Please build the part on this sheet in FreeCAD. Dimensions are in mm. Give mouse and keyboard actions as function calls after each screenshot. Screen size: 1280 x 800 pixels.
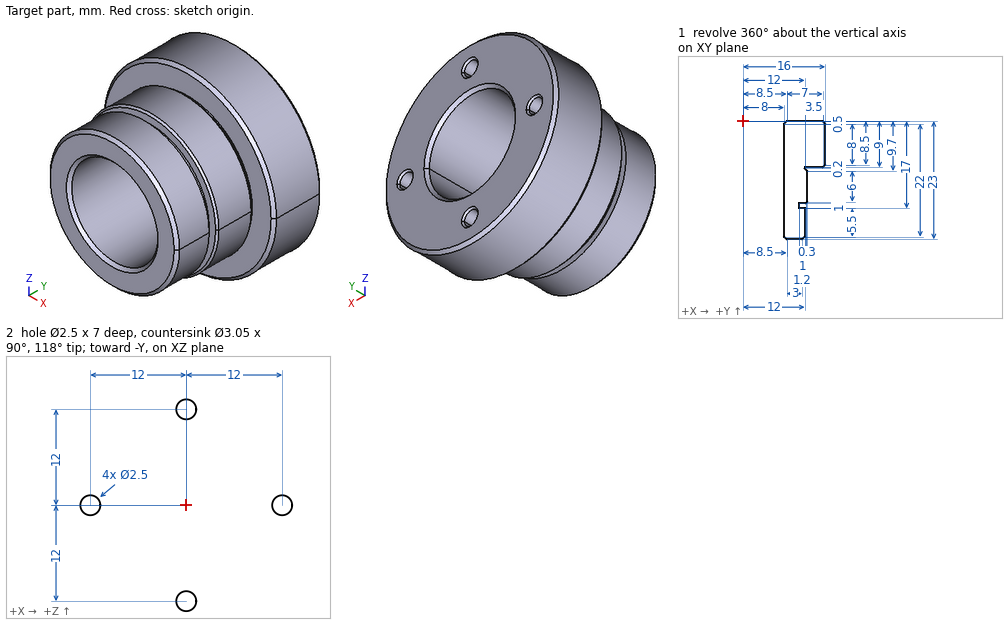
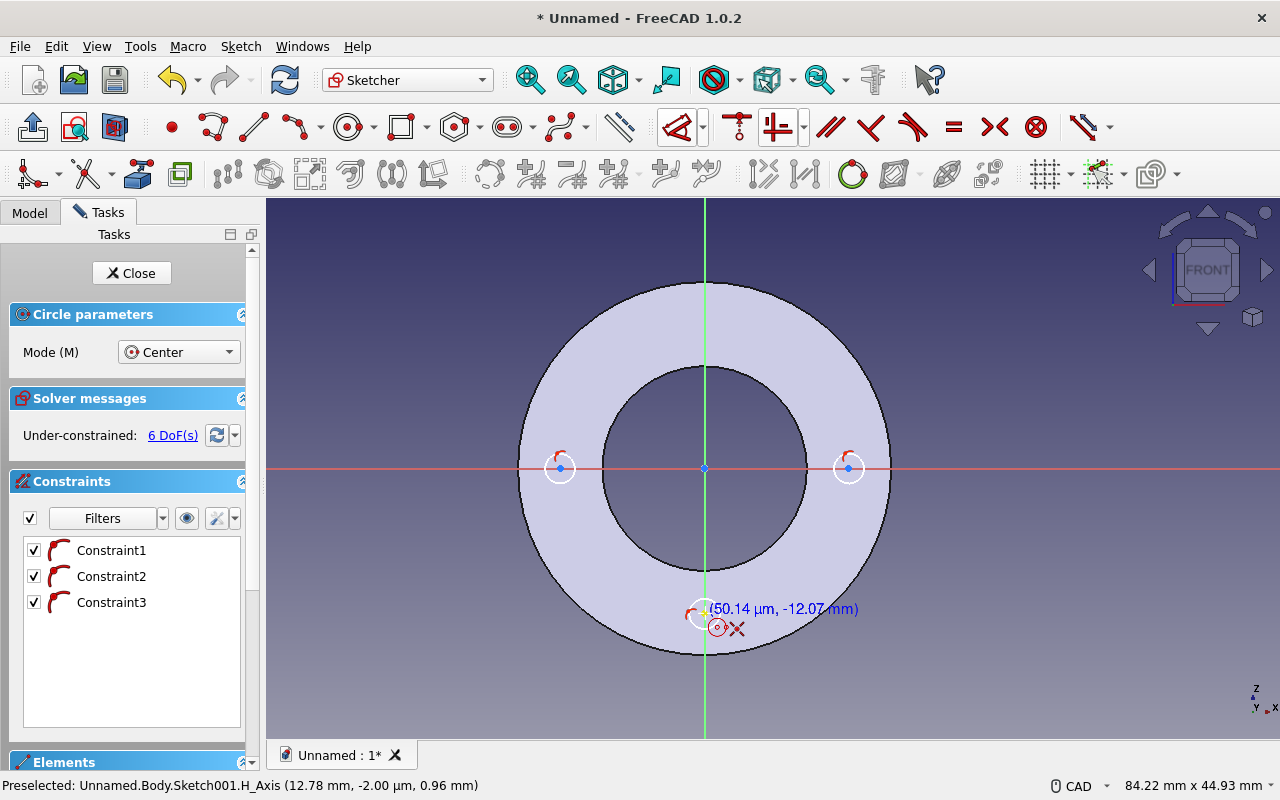
scroll(705, 324, up, 3)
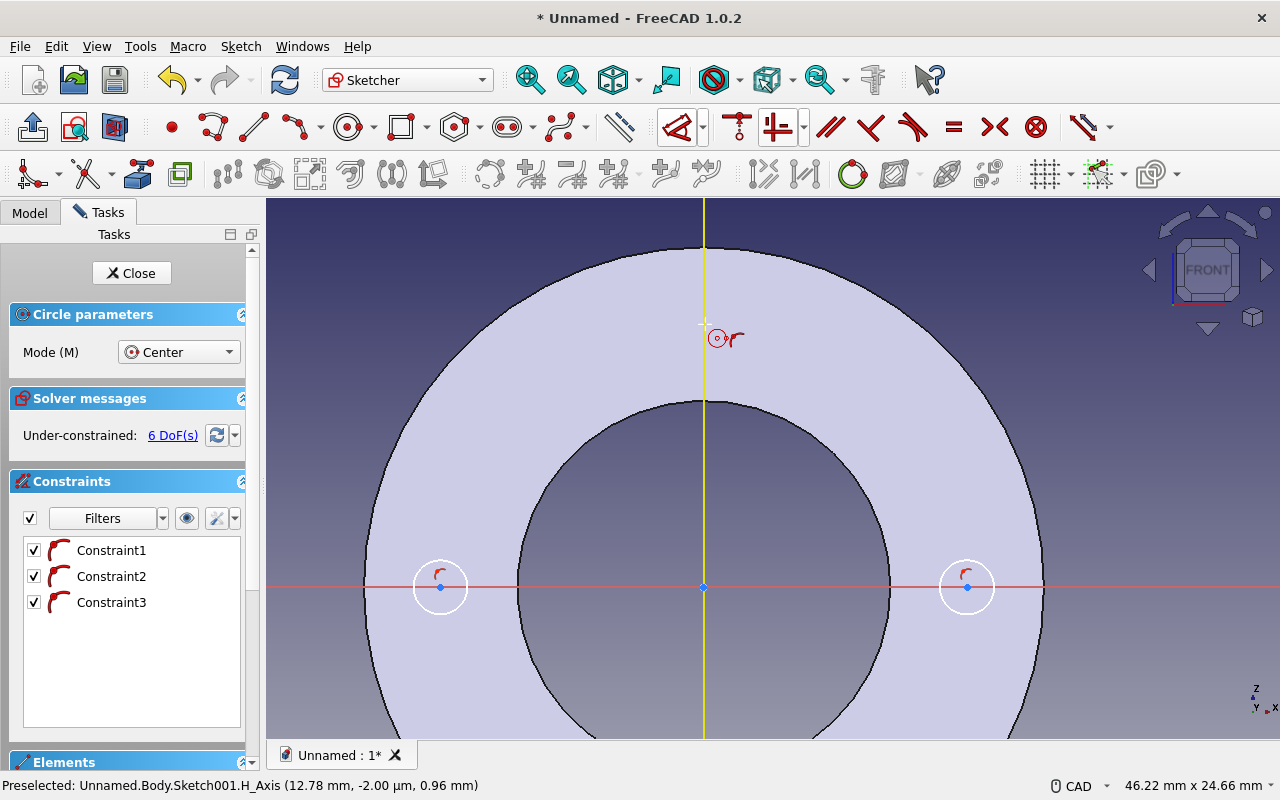
click(704, 324)
click(723, 305)
key(Escape)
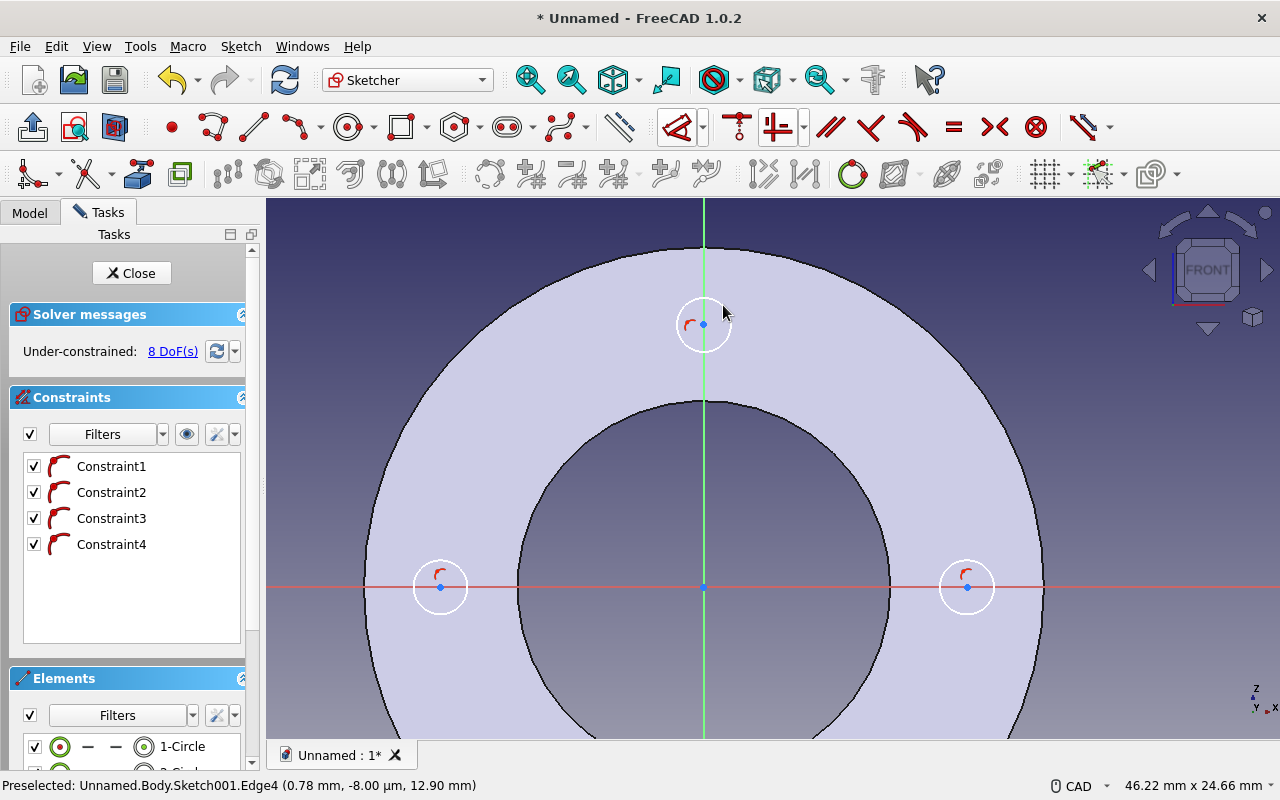
click(460, 568)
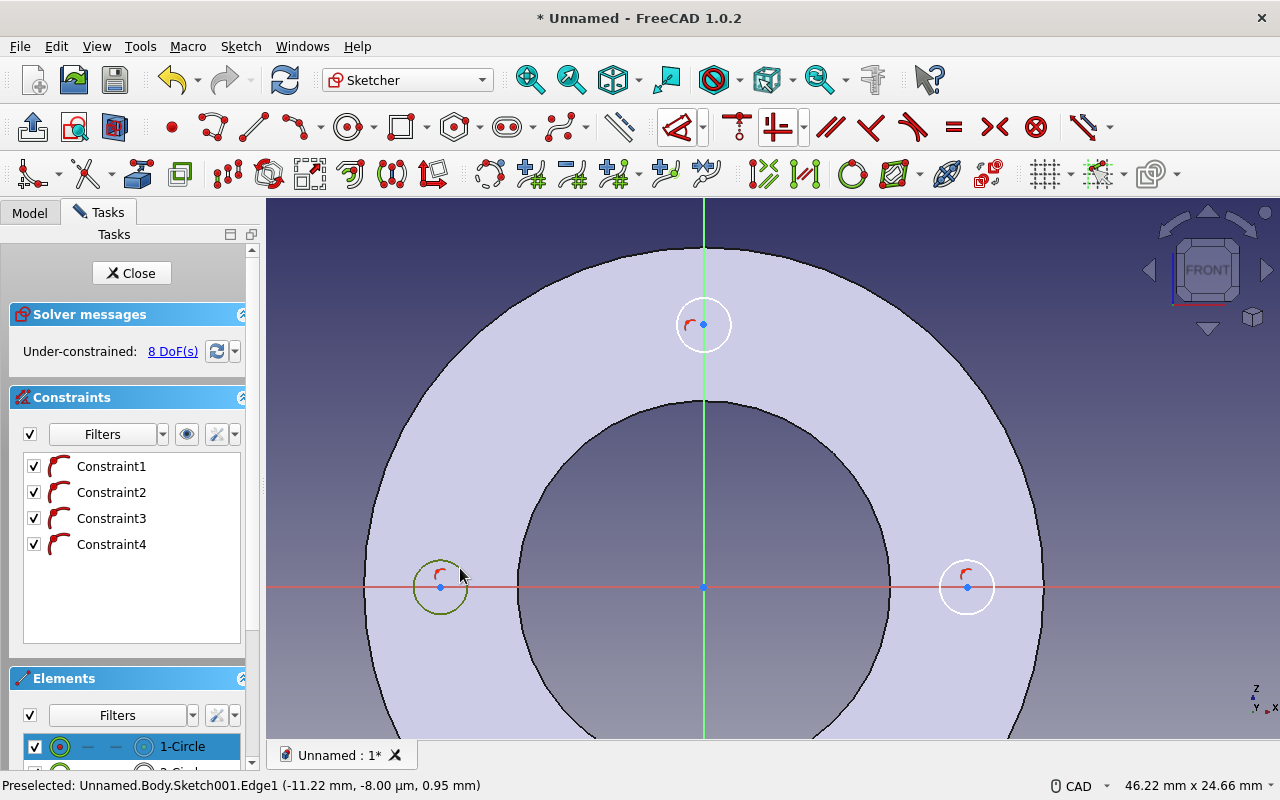
scroll(705, 324, down, 3)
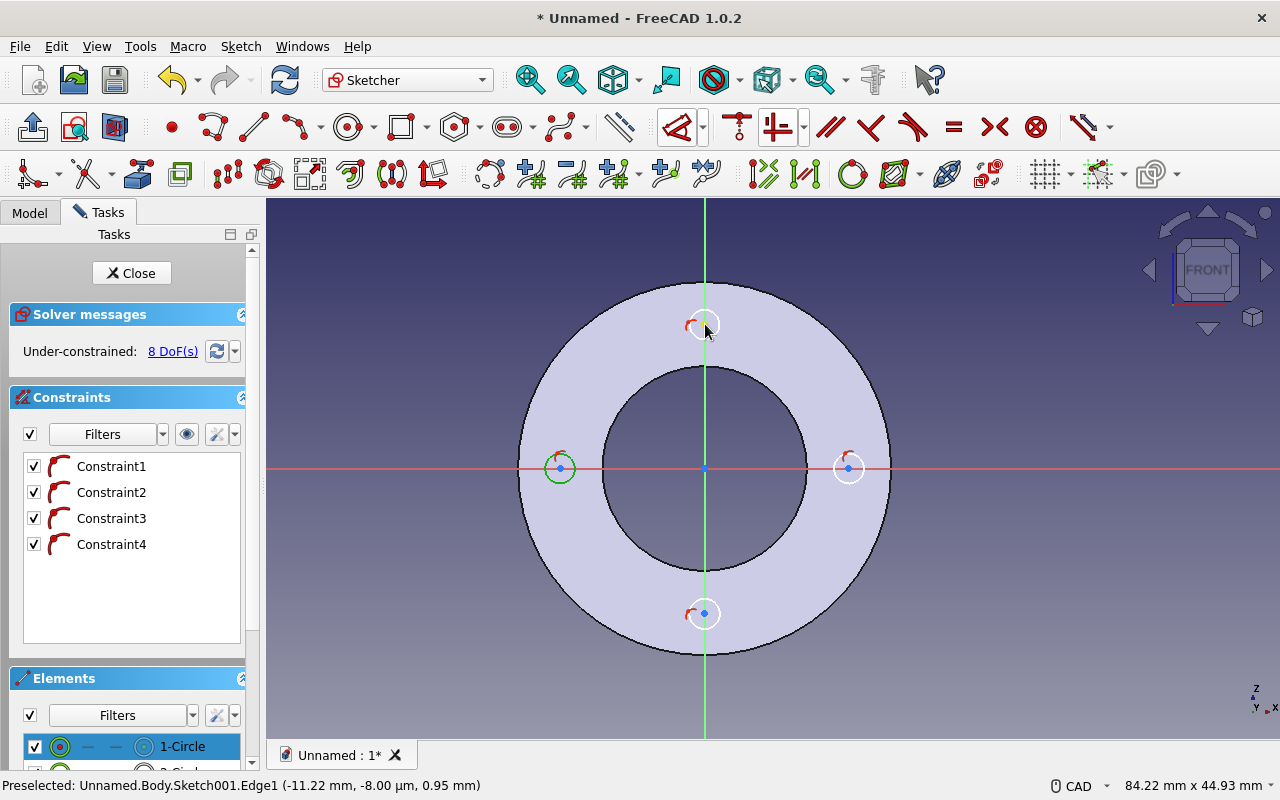
scroll(715, 603, up, 2)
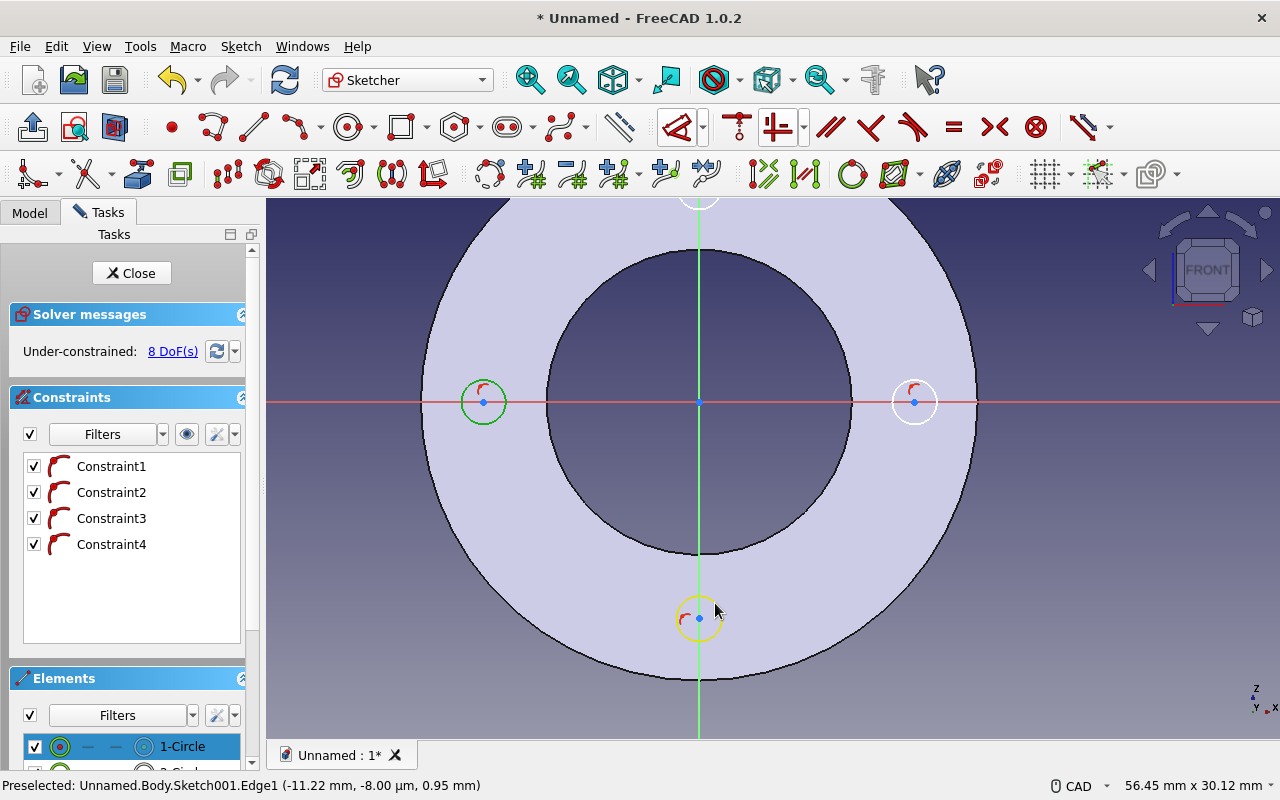
click(715, 603)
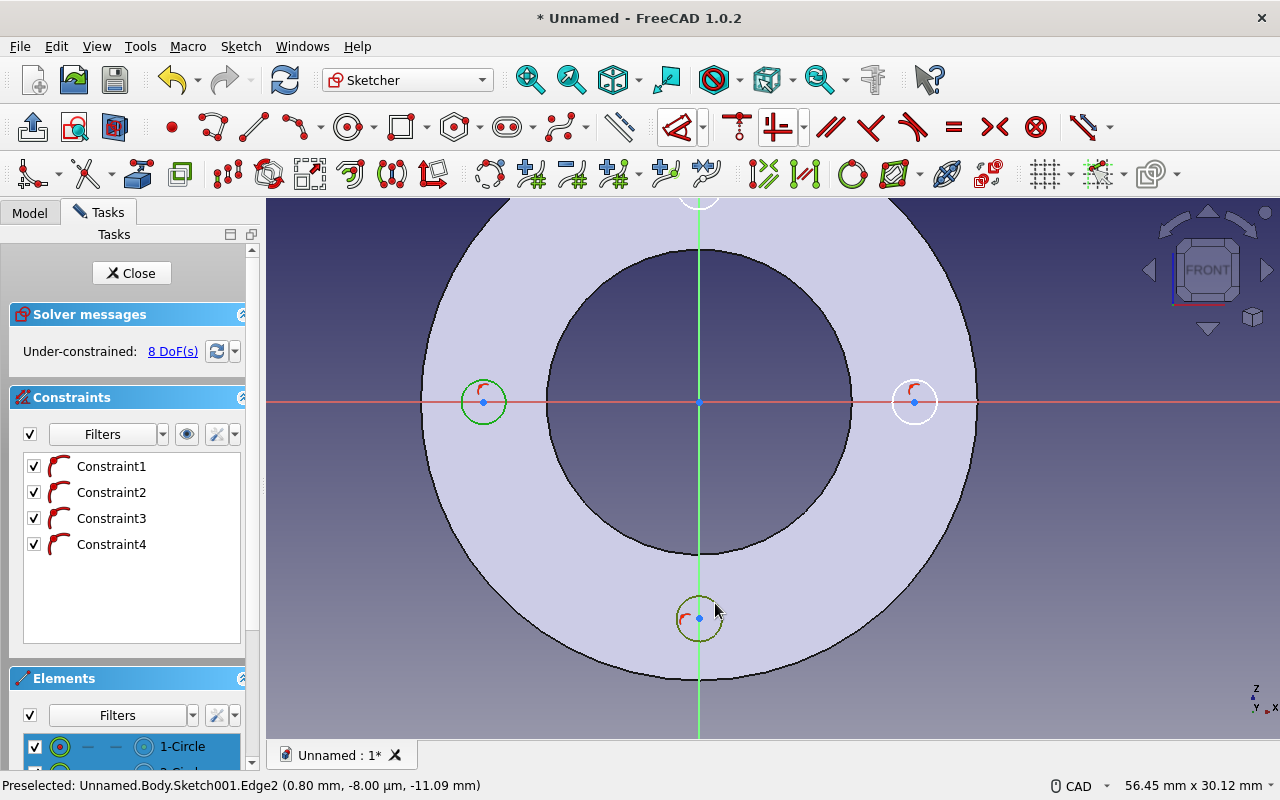
click(930, 386)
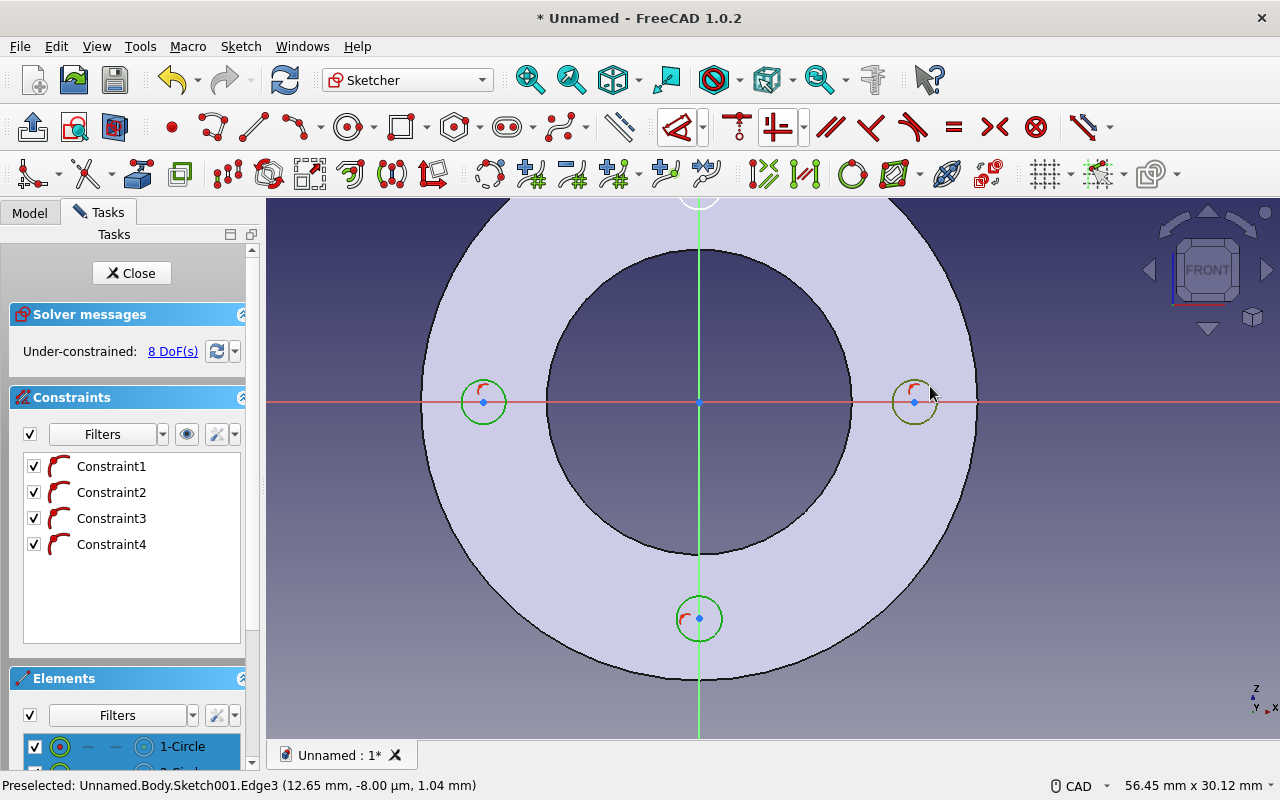
scroll(715, 603, down, 2)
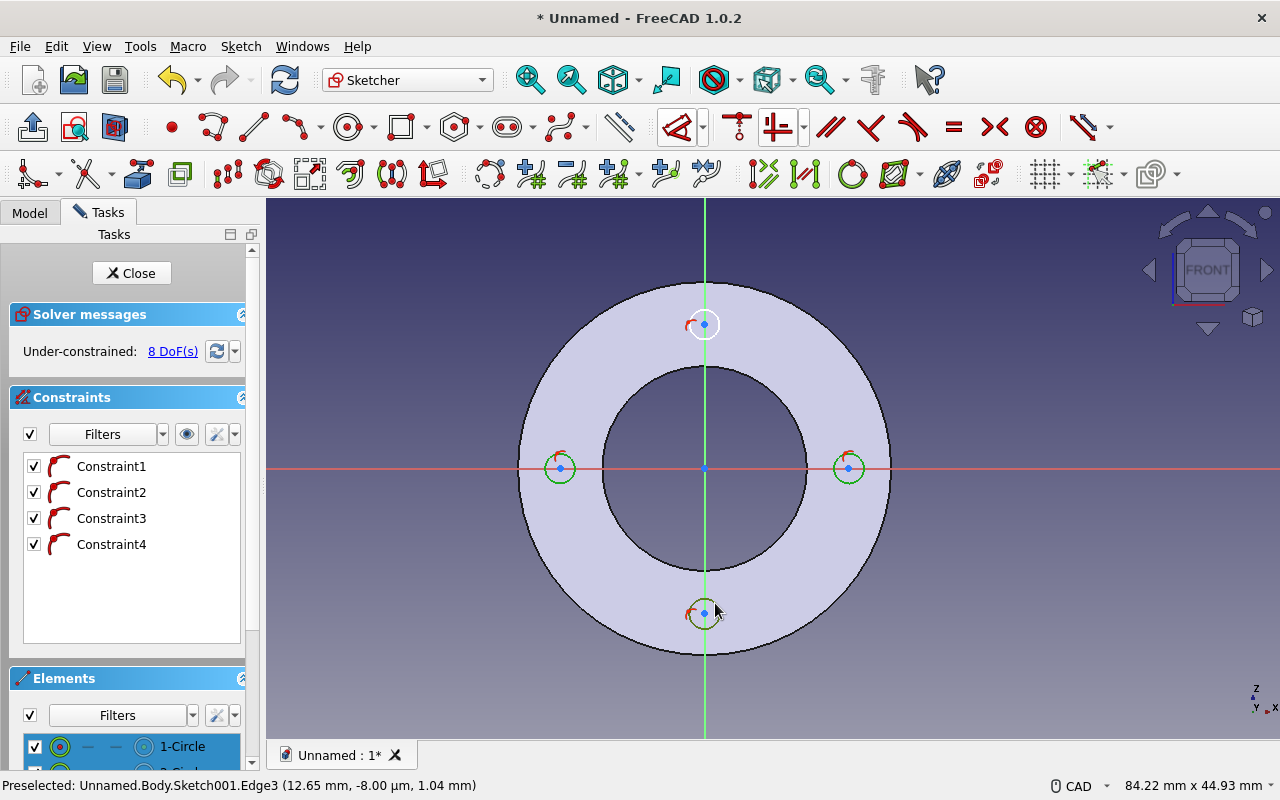
scroll(715, 314, up, 2)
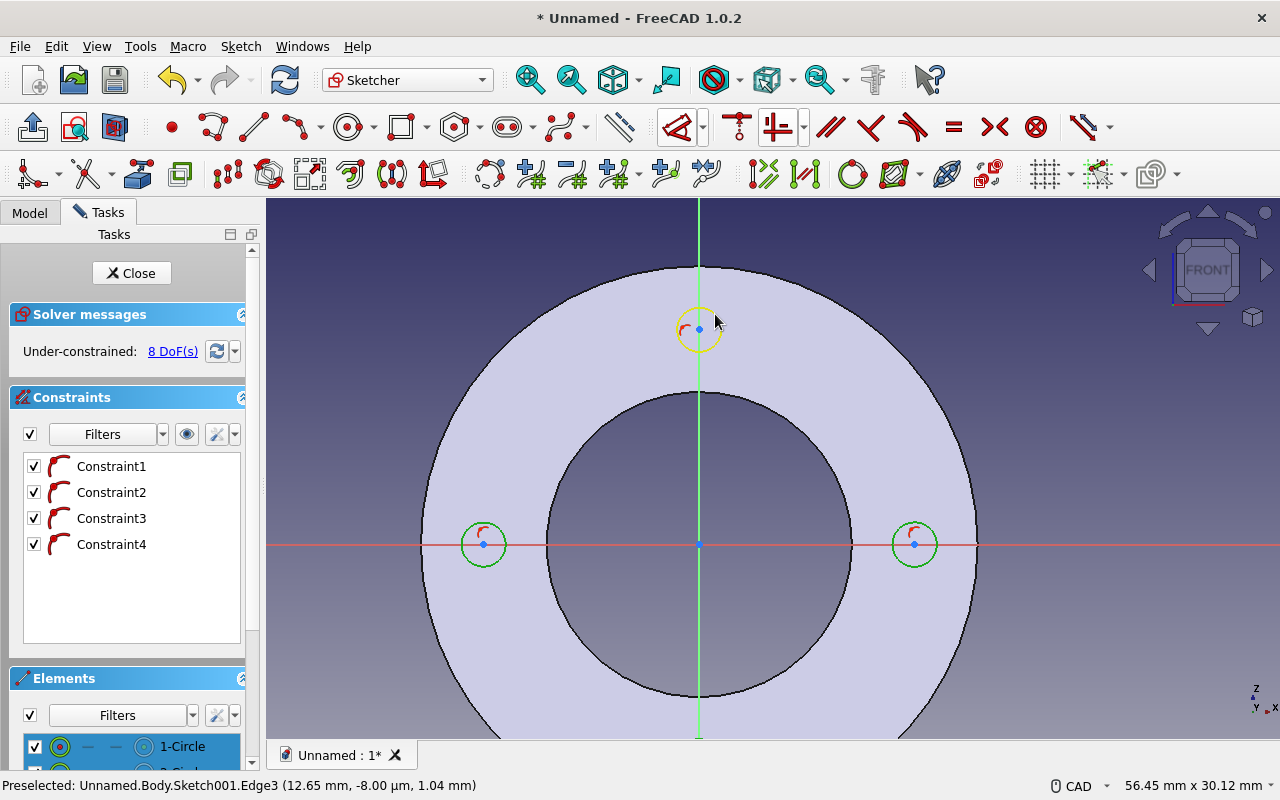
click(715, 314)